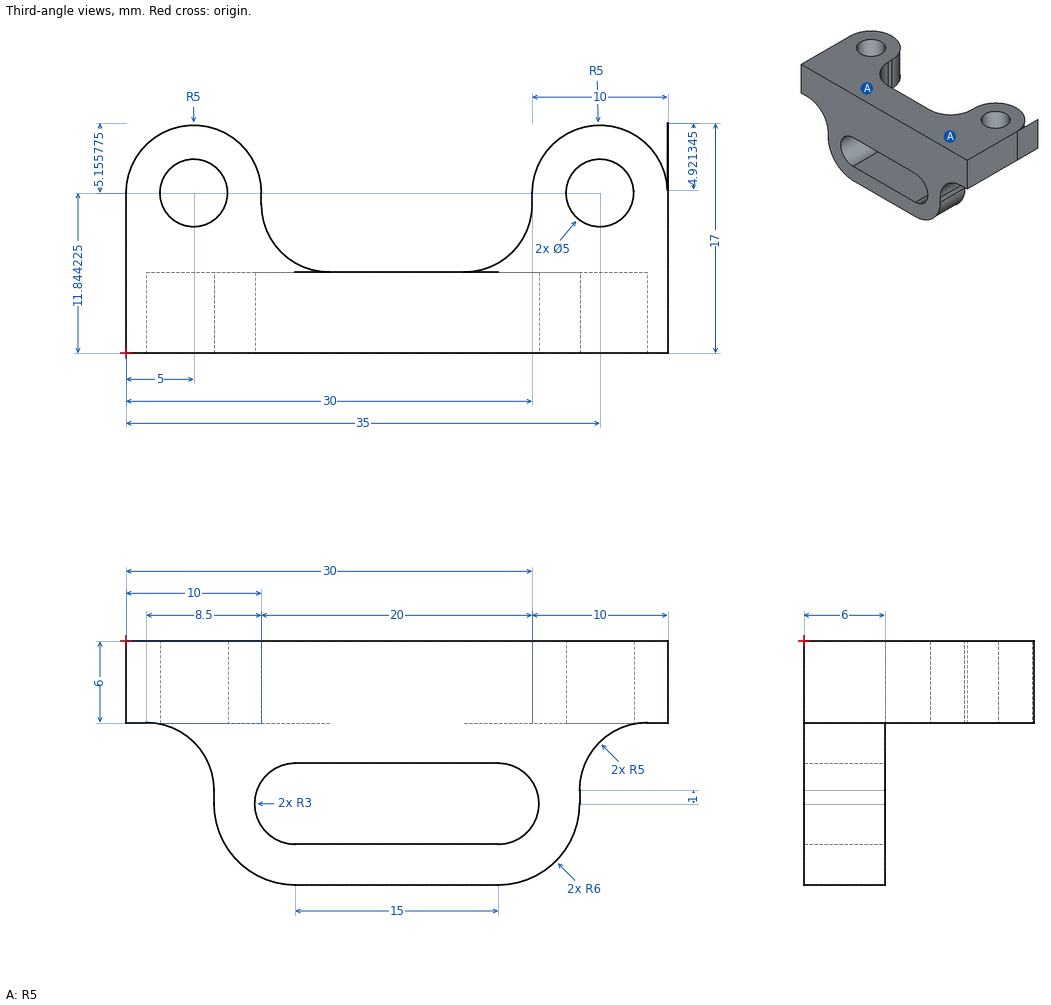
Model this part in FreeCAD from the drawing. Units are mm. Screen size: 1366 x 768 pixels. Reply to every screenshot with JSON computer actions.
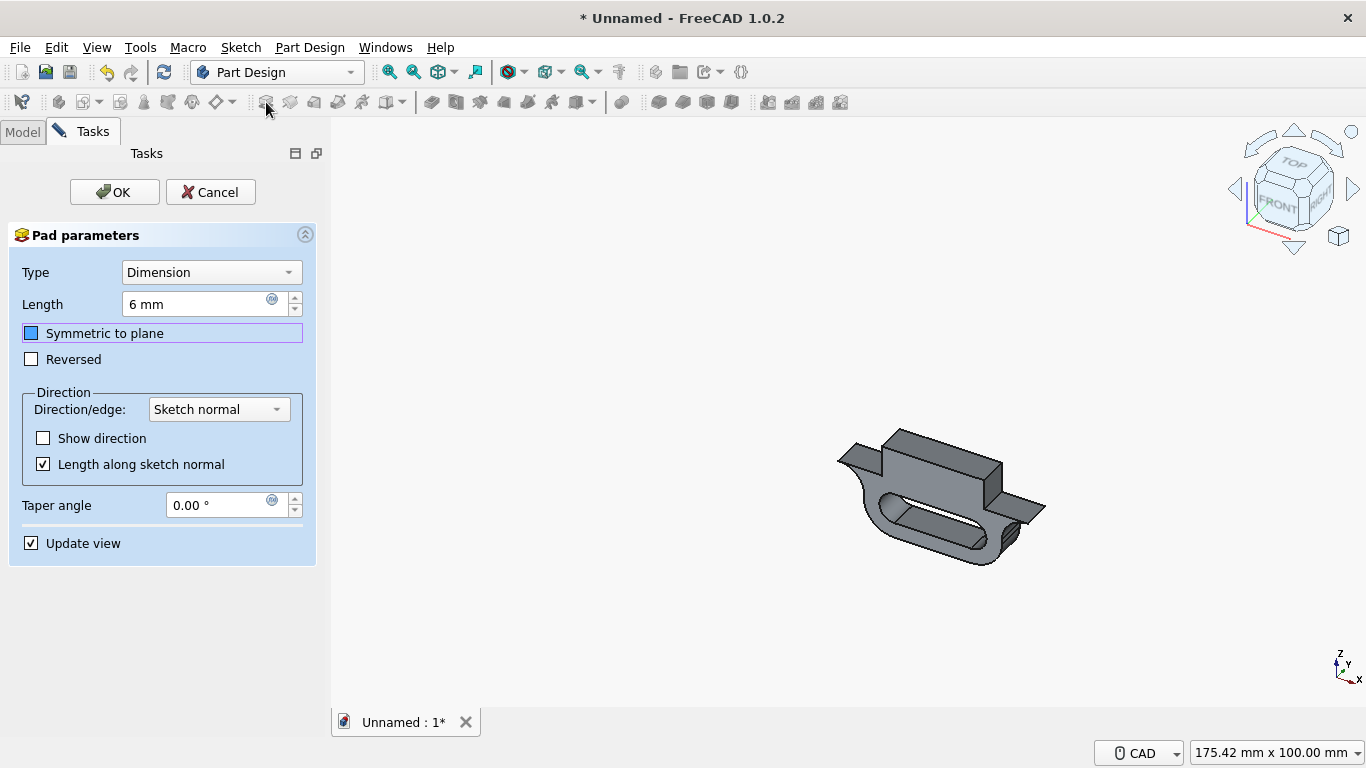
{"action": "left_click", "coordinate": [30, 359]}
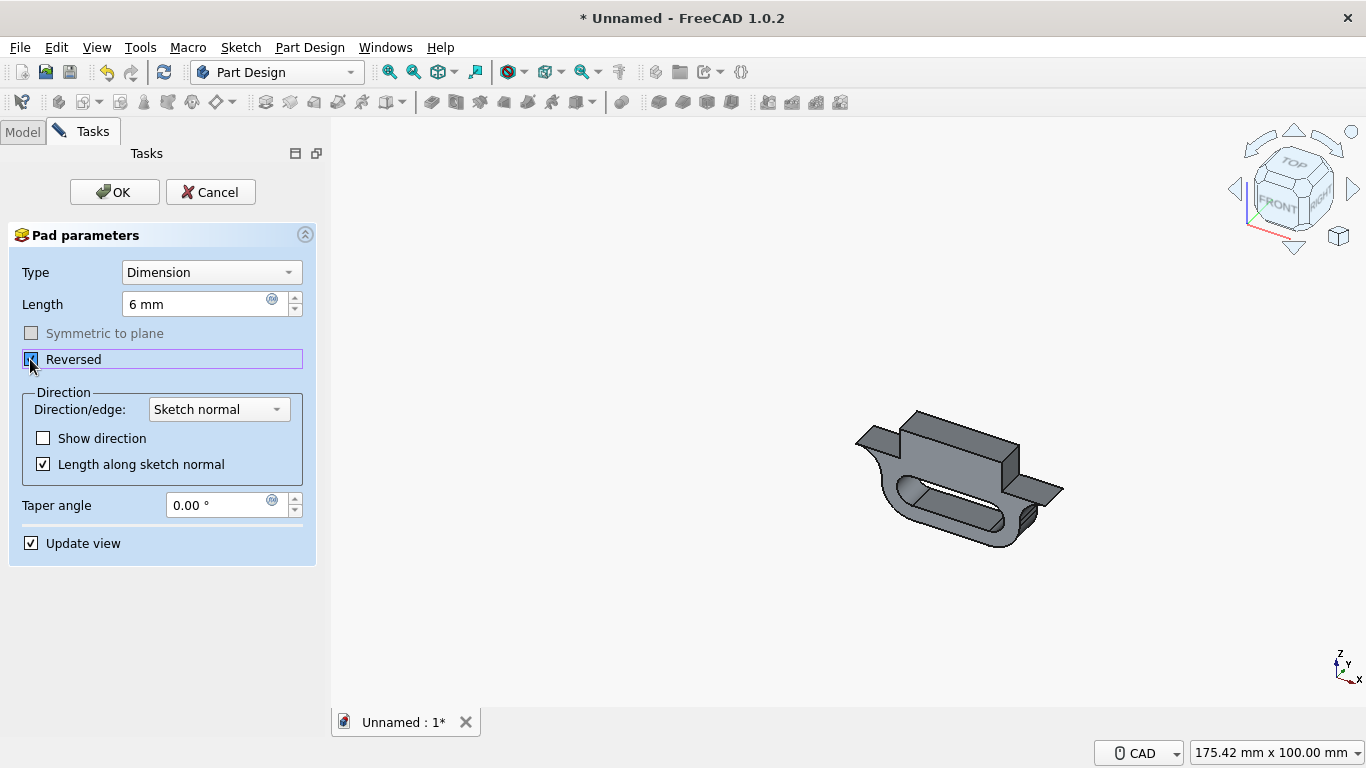
{"action": "left_click", "coordinate": [115, 192]}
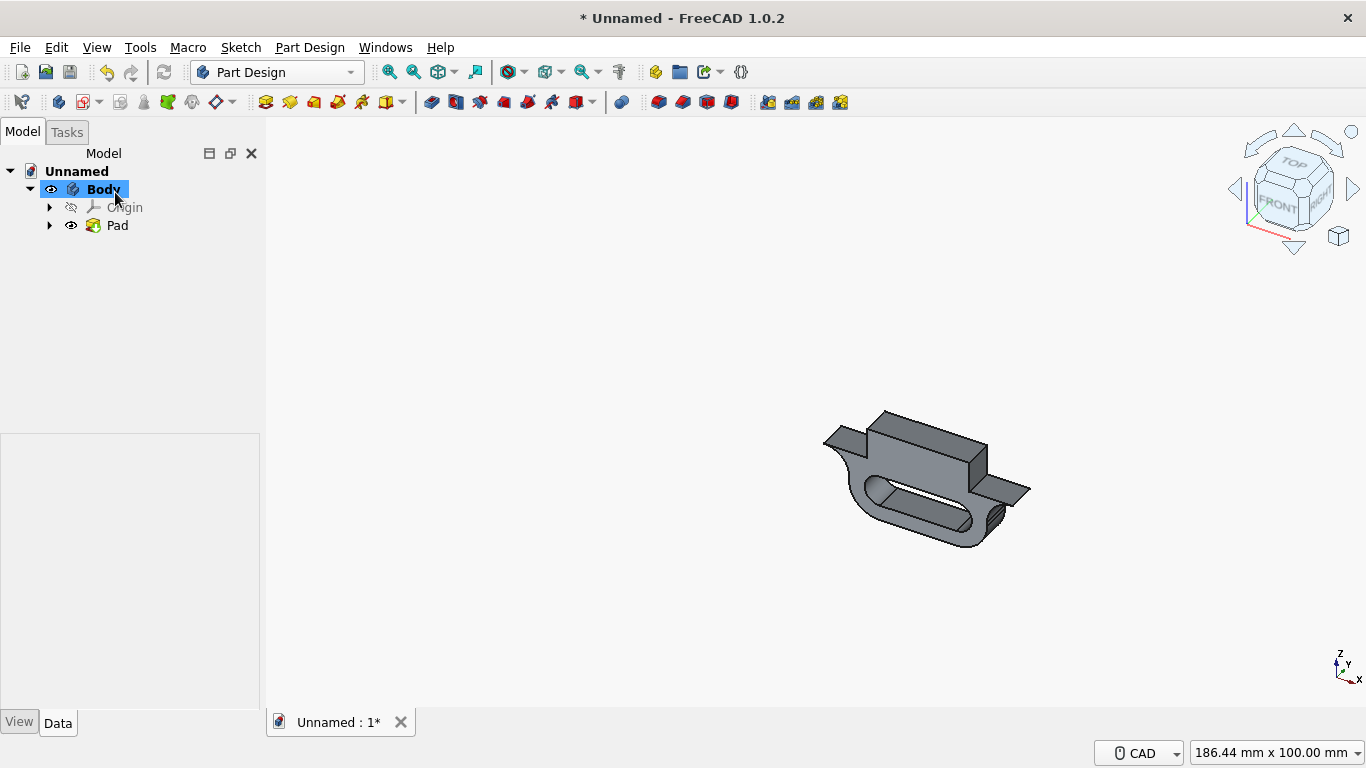
{"action": "key", "text": "v f"}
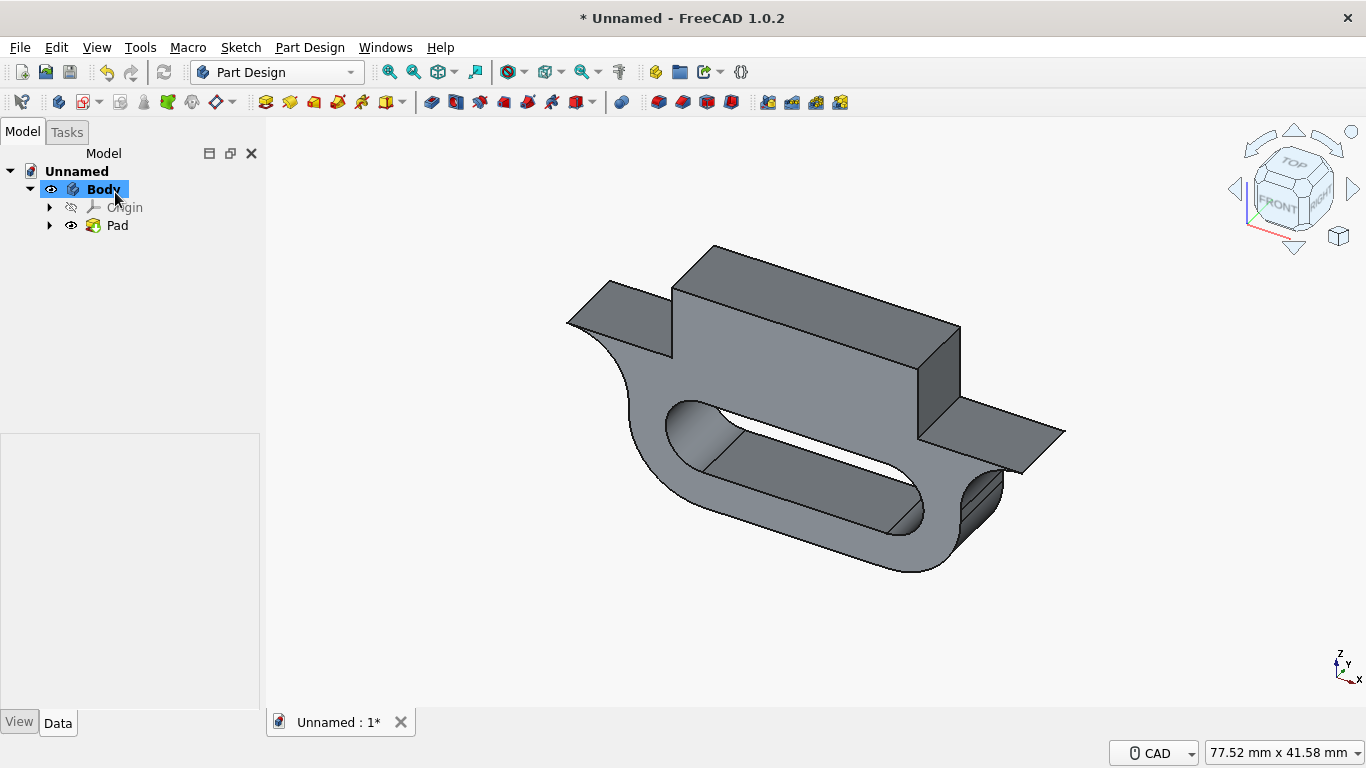
{"action": "left_click", "coordinate": [84, 102]}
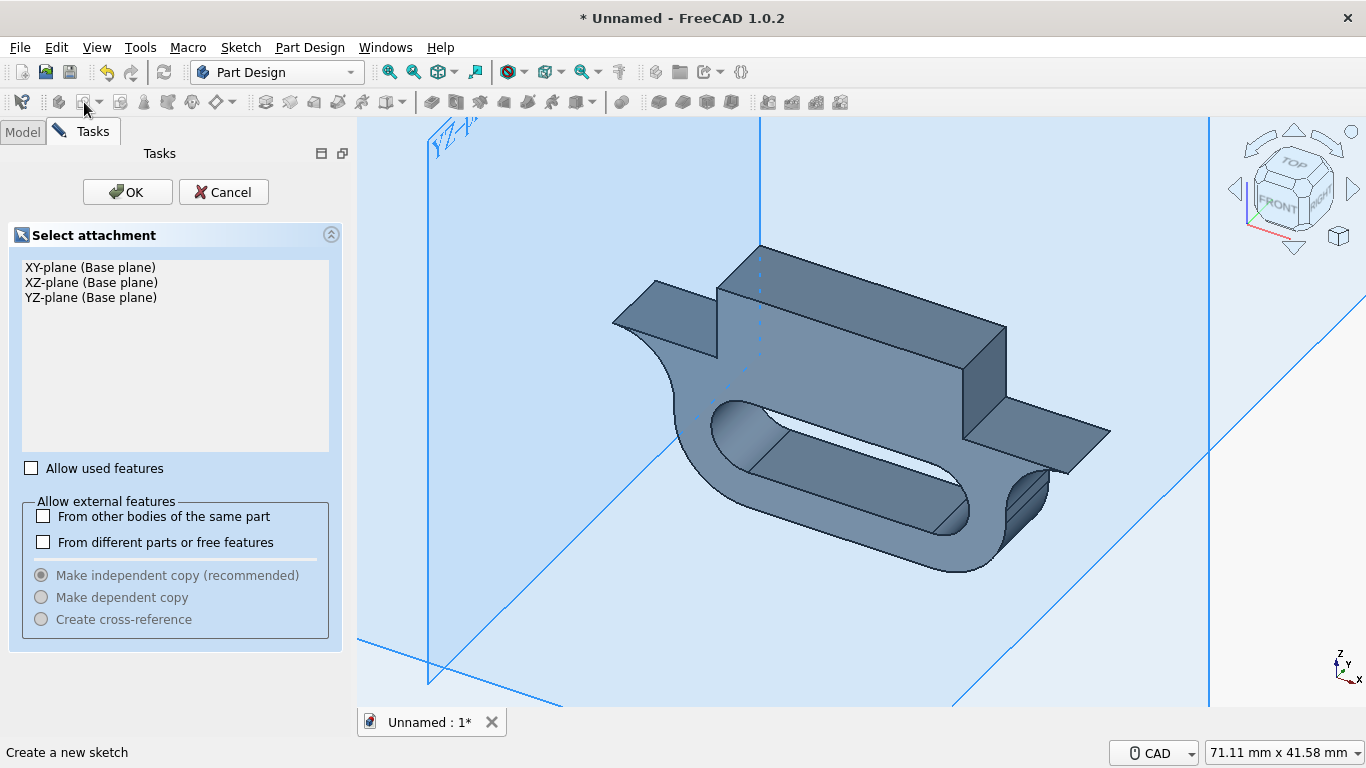
{"action": "left_click", "coordinate": [82, 282]}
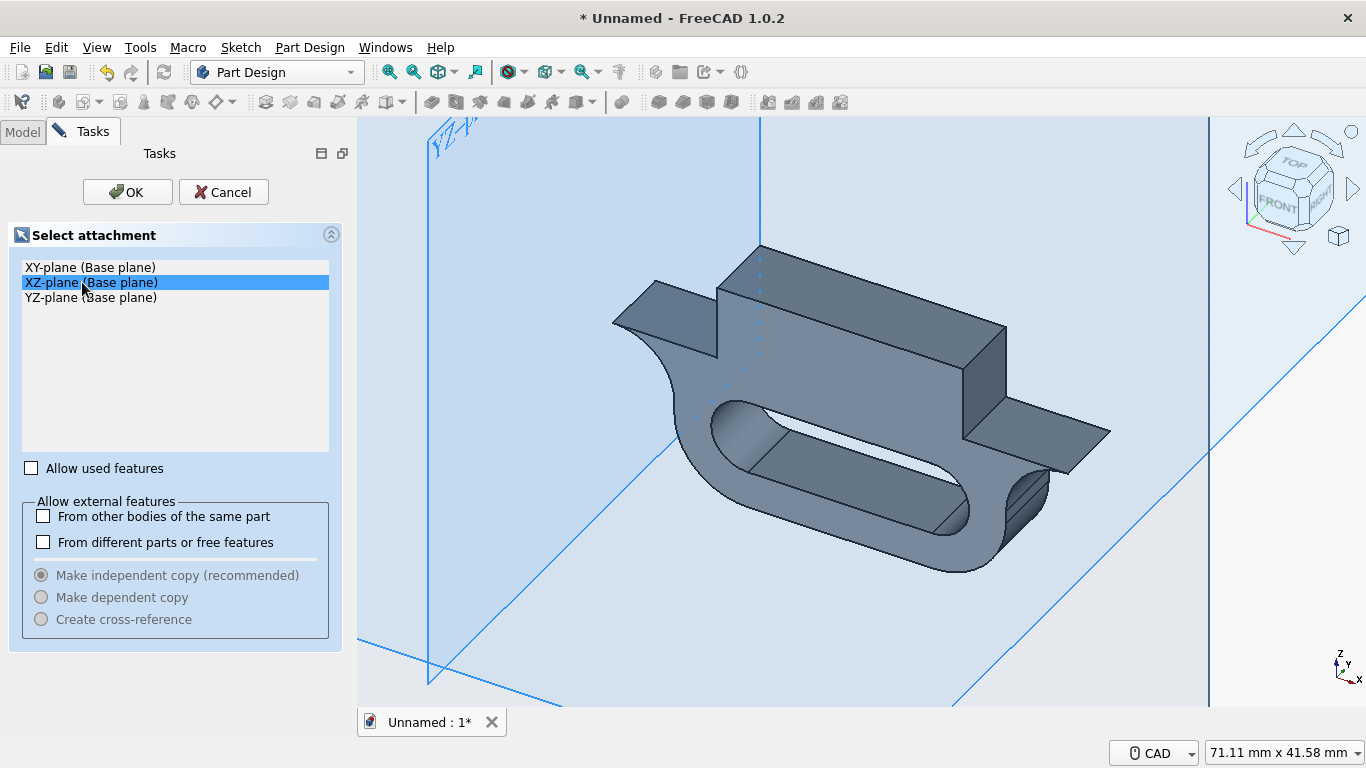
{"action": "left_click", "coordinate": [128, 192]}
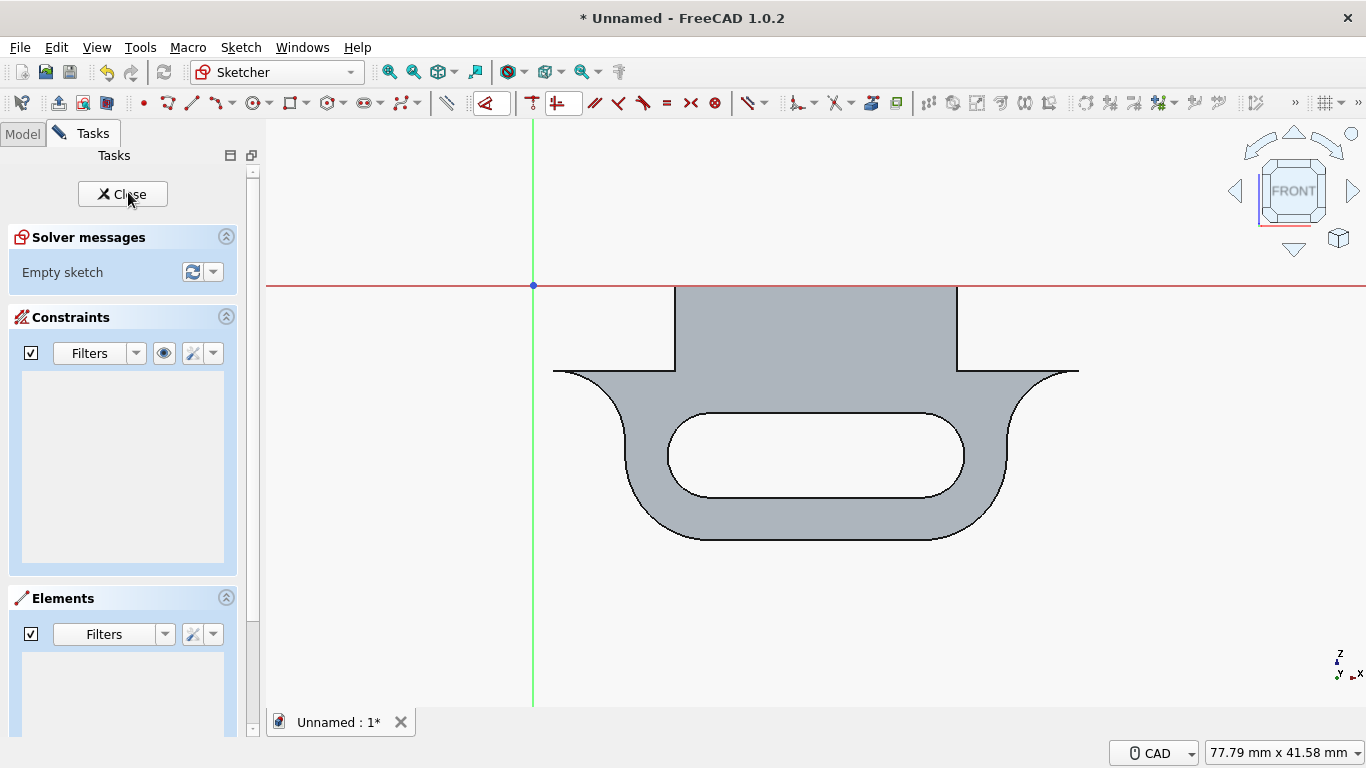
{"action": "left_click", "coordinate": [290, 104]}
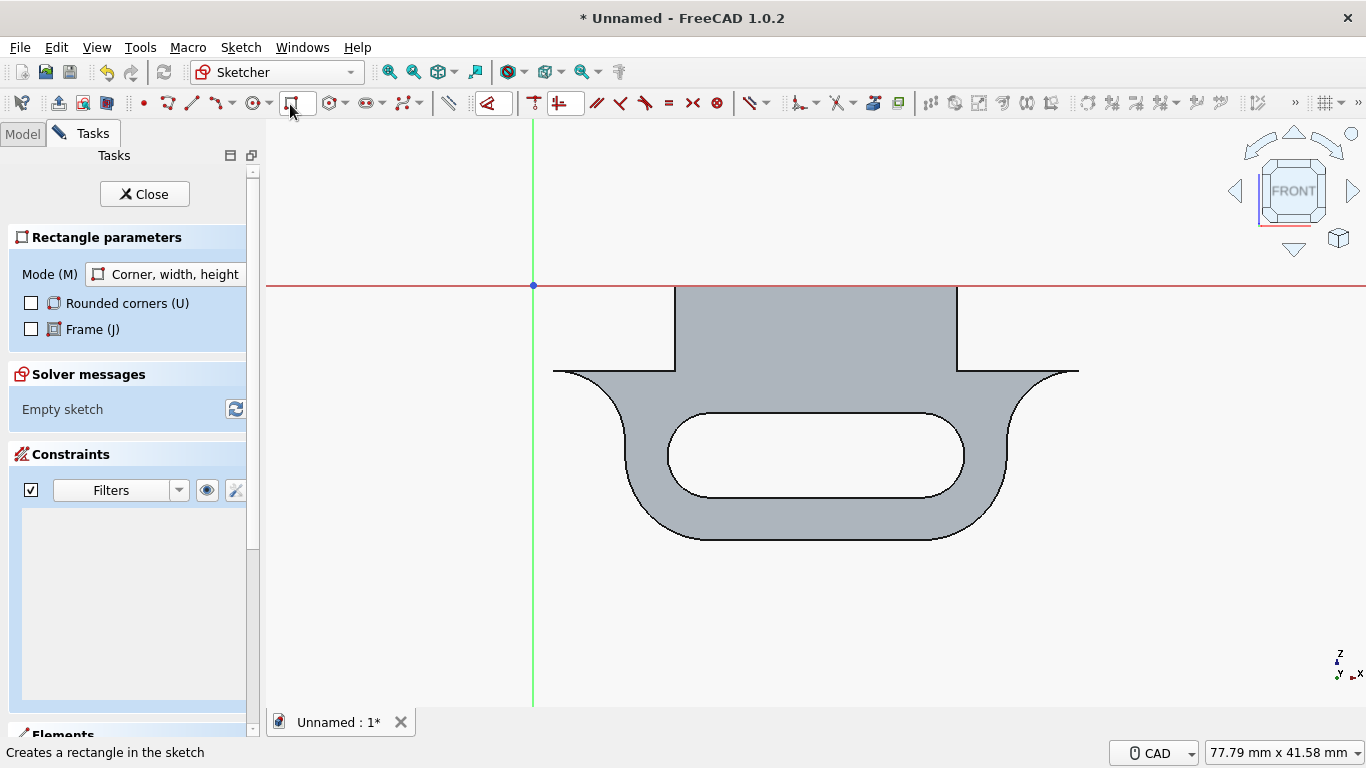
{"action": "left_click", "coordinate": [957, 286]}
{"action": "mouse_move", "coordinate": [1099, 371]}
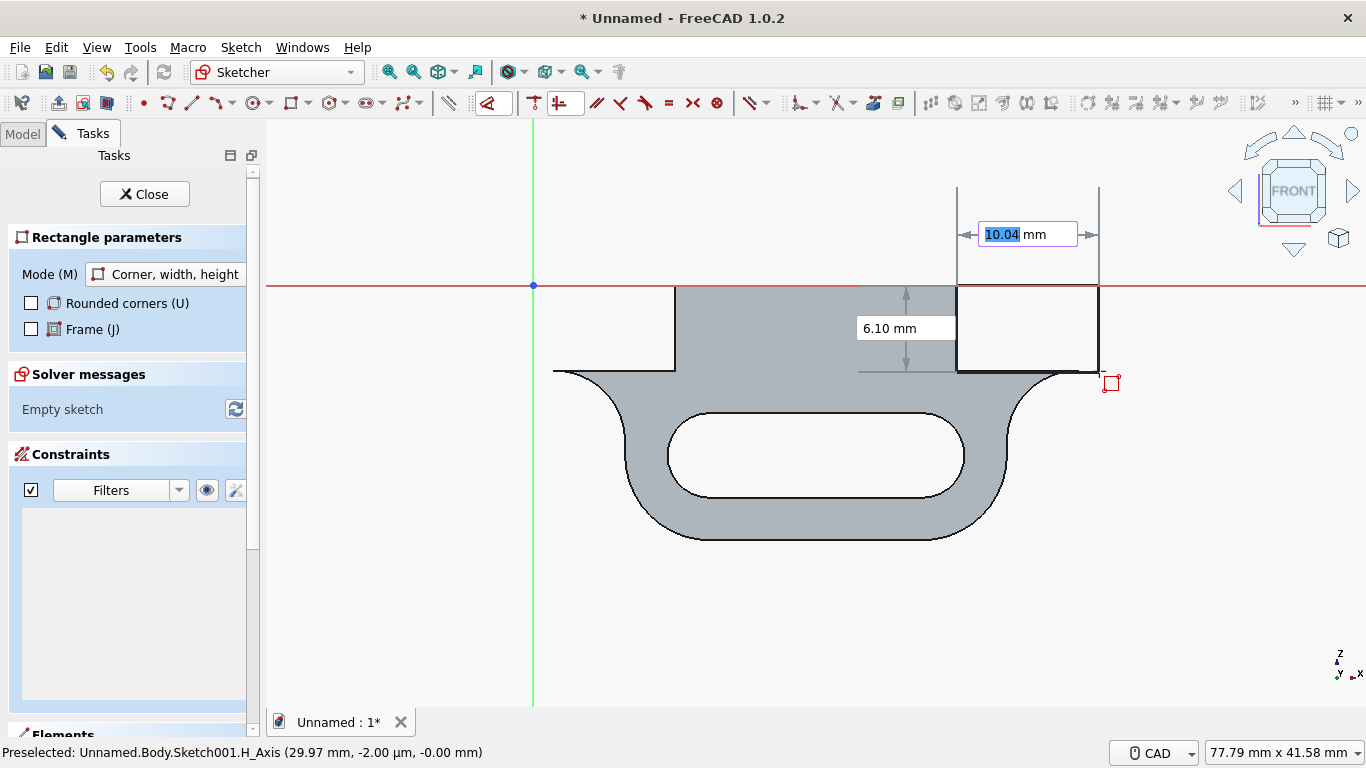
{"action": "type", "text": "10"}
{"action": "key", "text": "Tab"}
{"action": "type", "text": "6"}
{"action": "key", "text": "Return"}